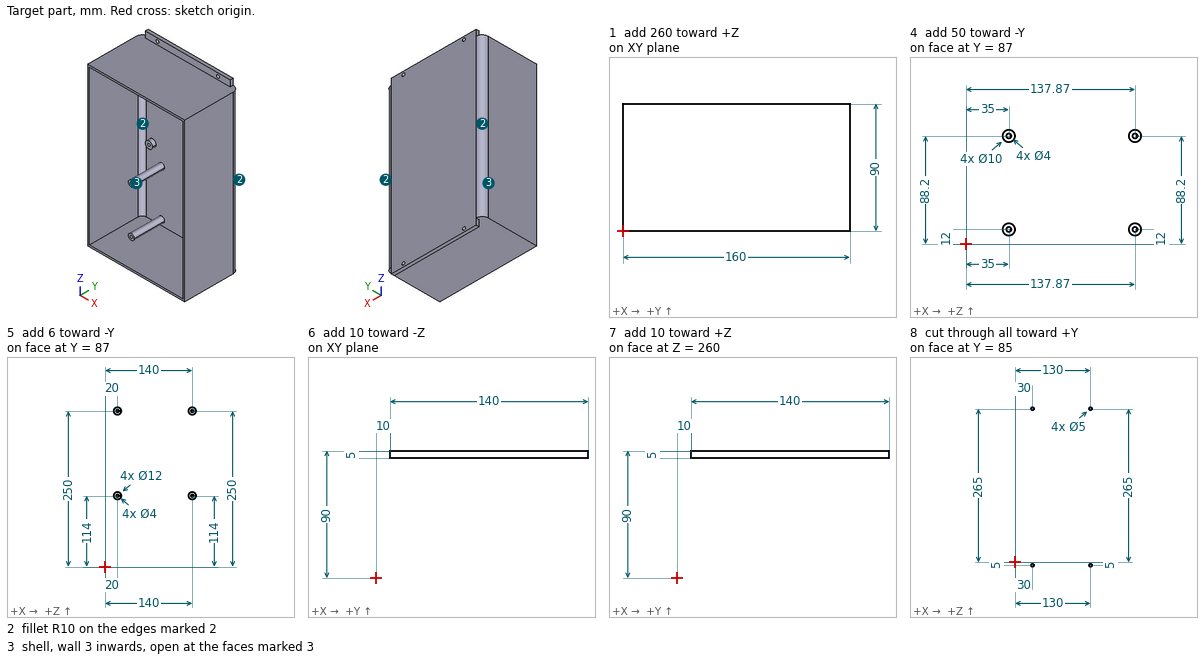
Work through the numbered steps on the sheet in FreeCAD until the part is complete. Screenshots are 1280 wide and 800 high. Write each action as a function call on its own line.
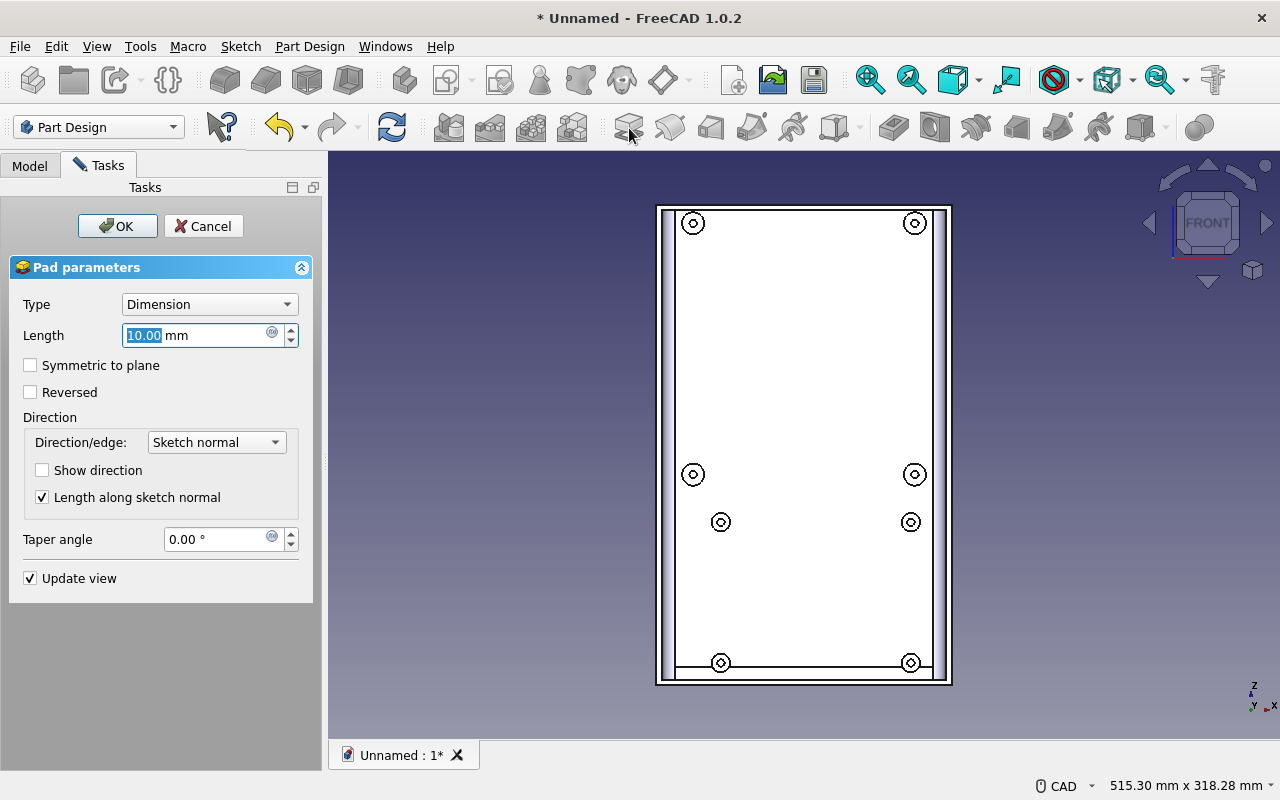
text(10)
key(Tab)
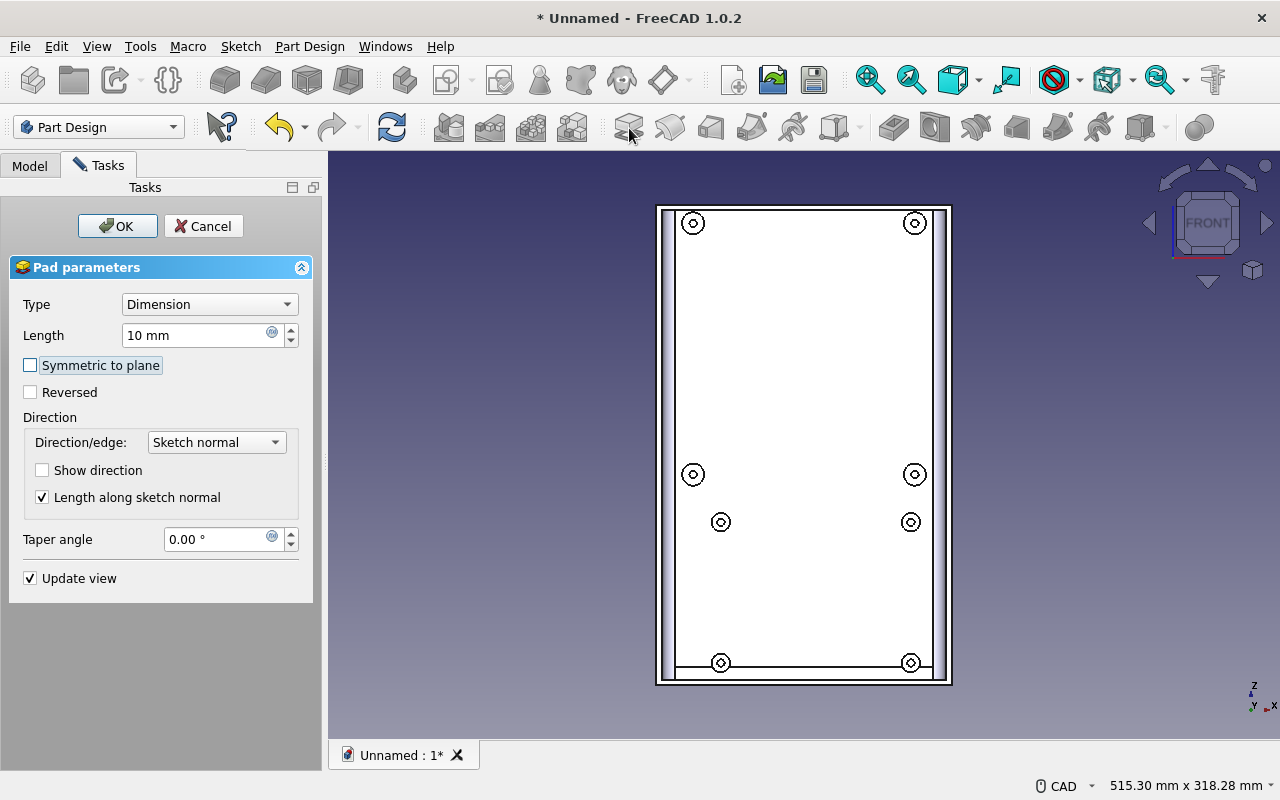
click(31, 392)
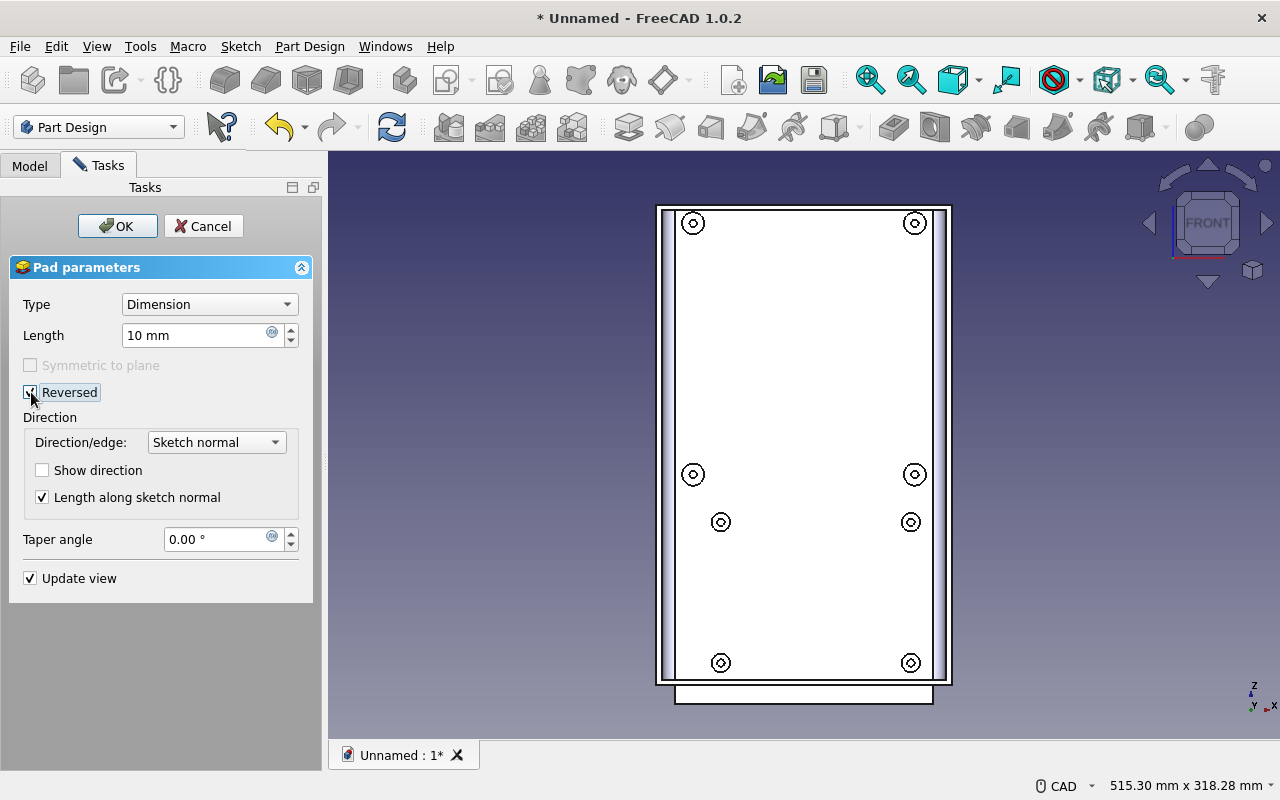
click(118, 226)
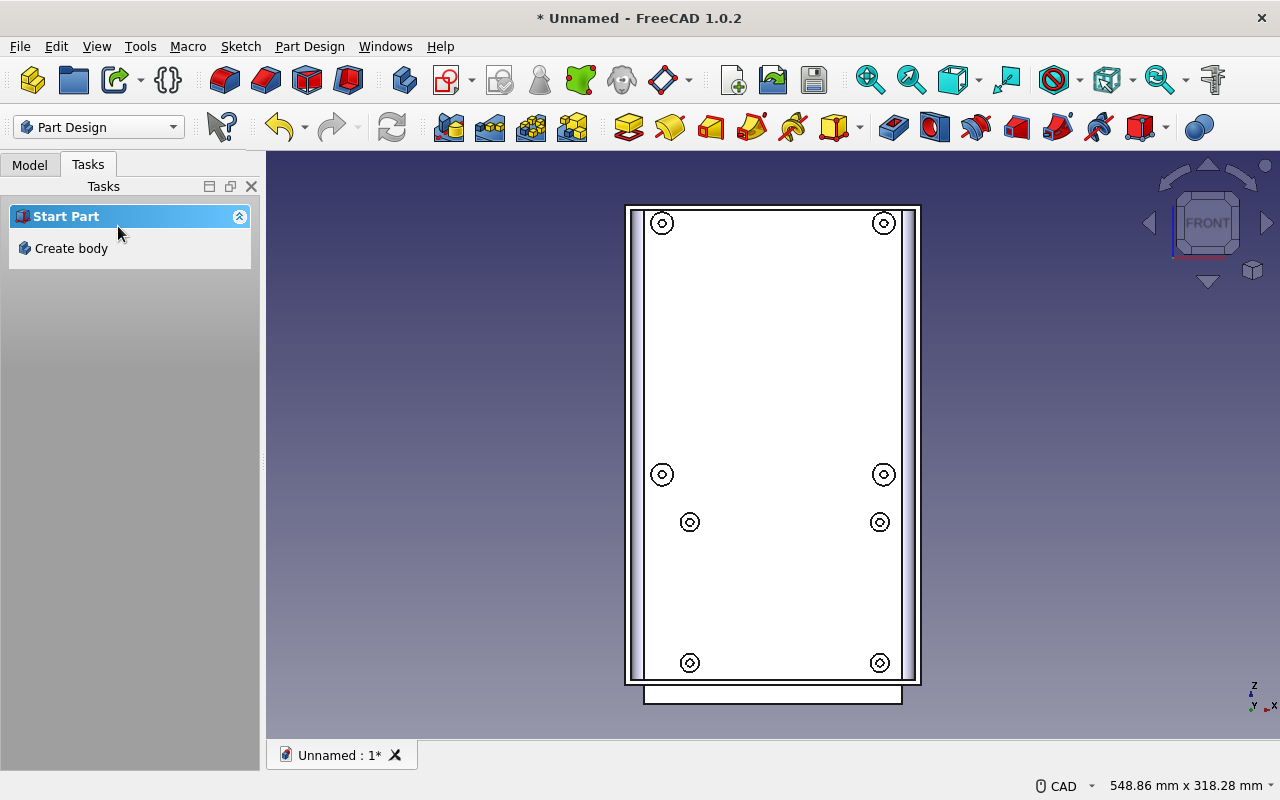
key(0)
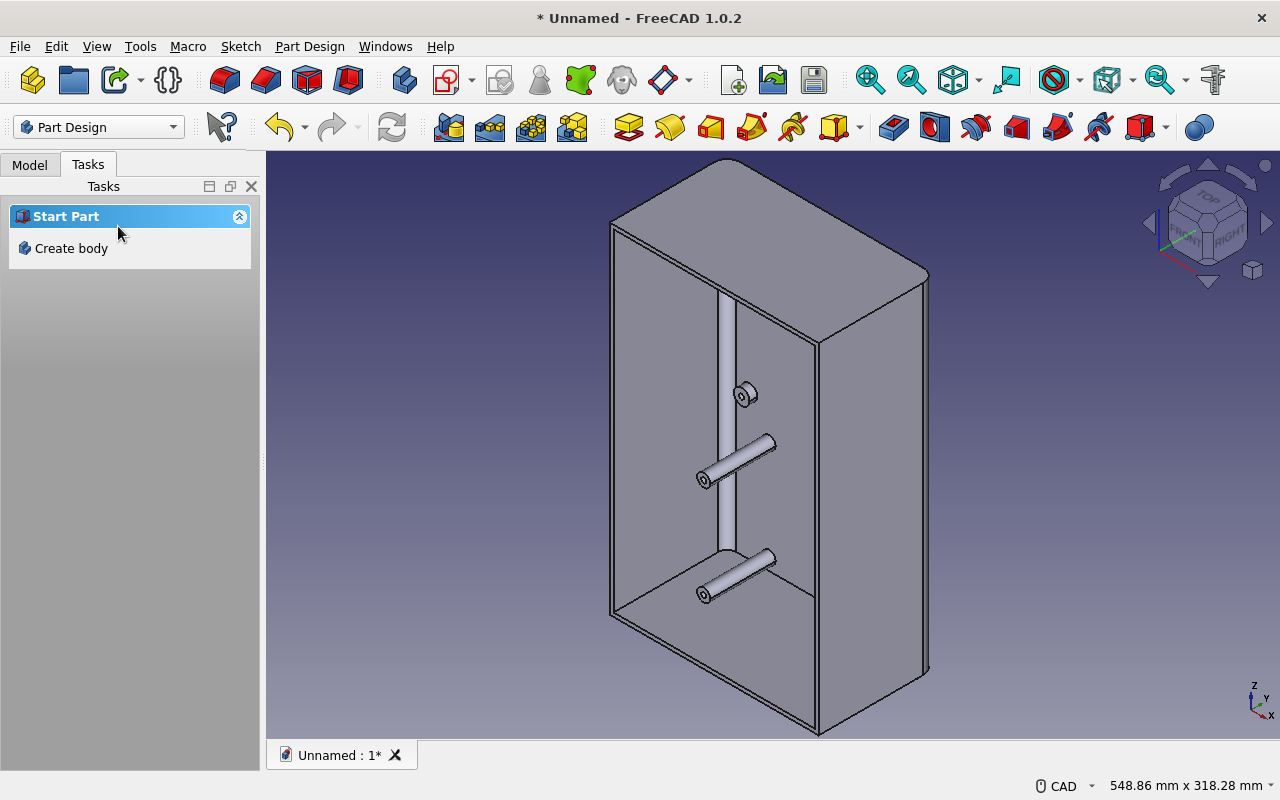
click(871, 80)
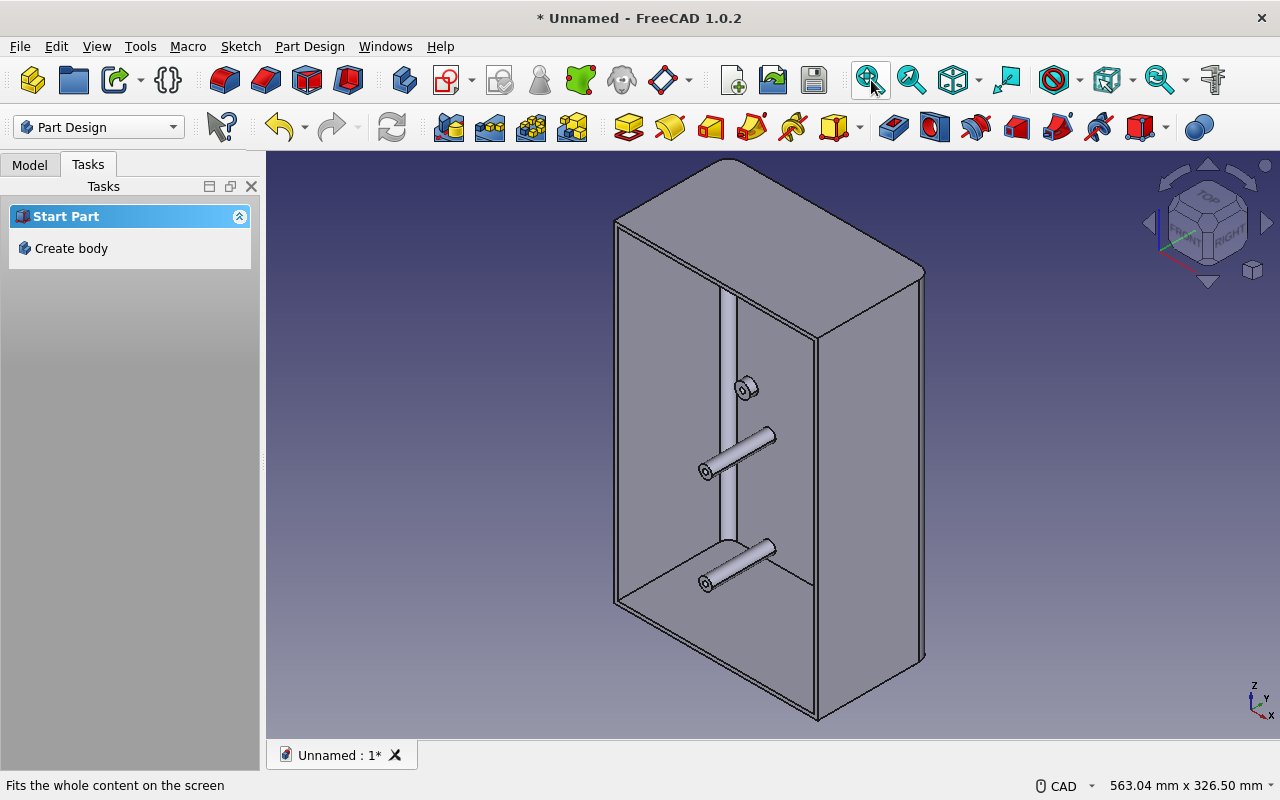
click(802, 262)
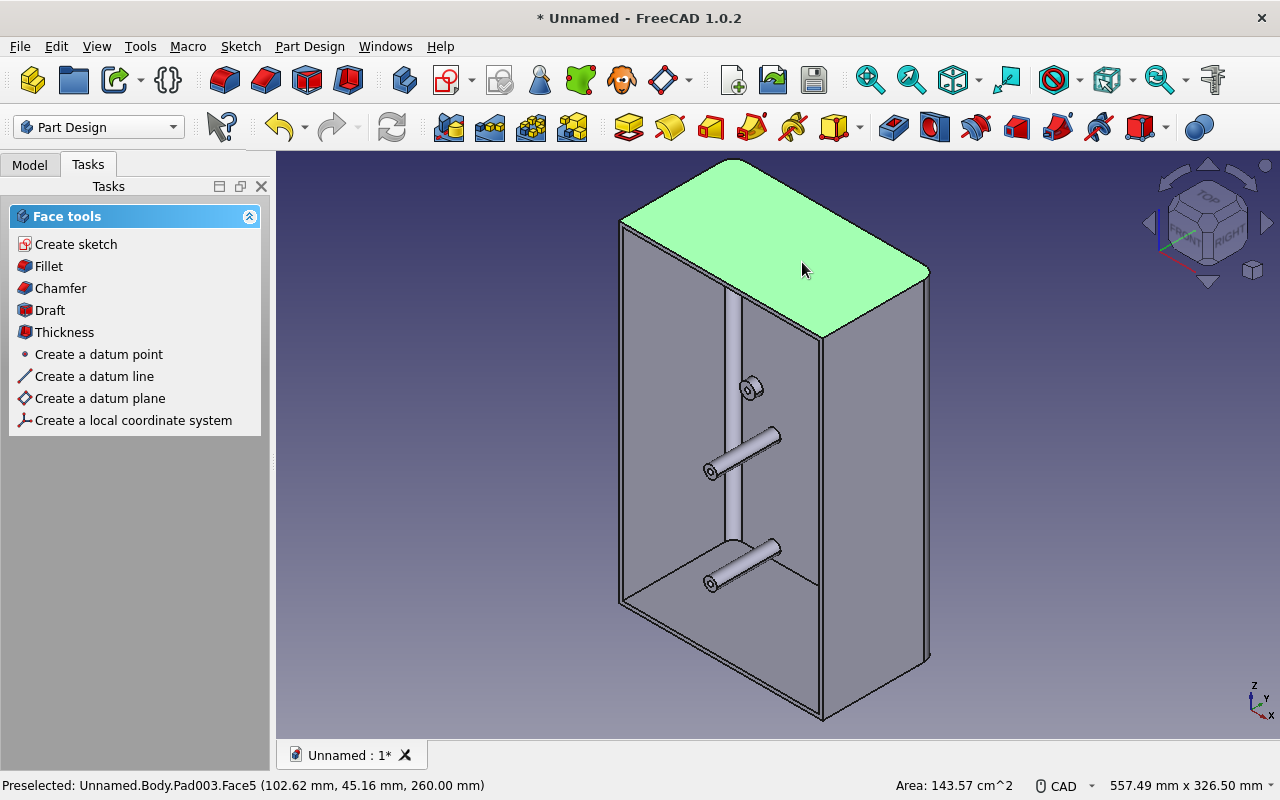
click(446, 80)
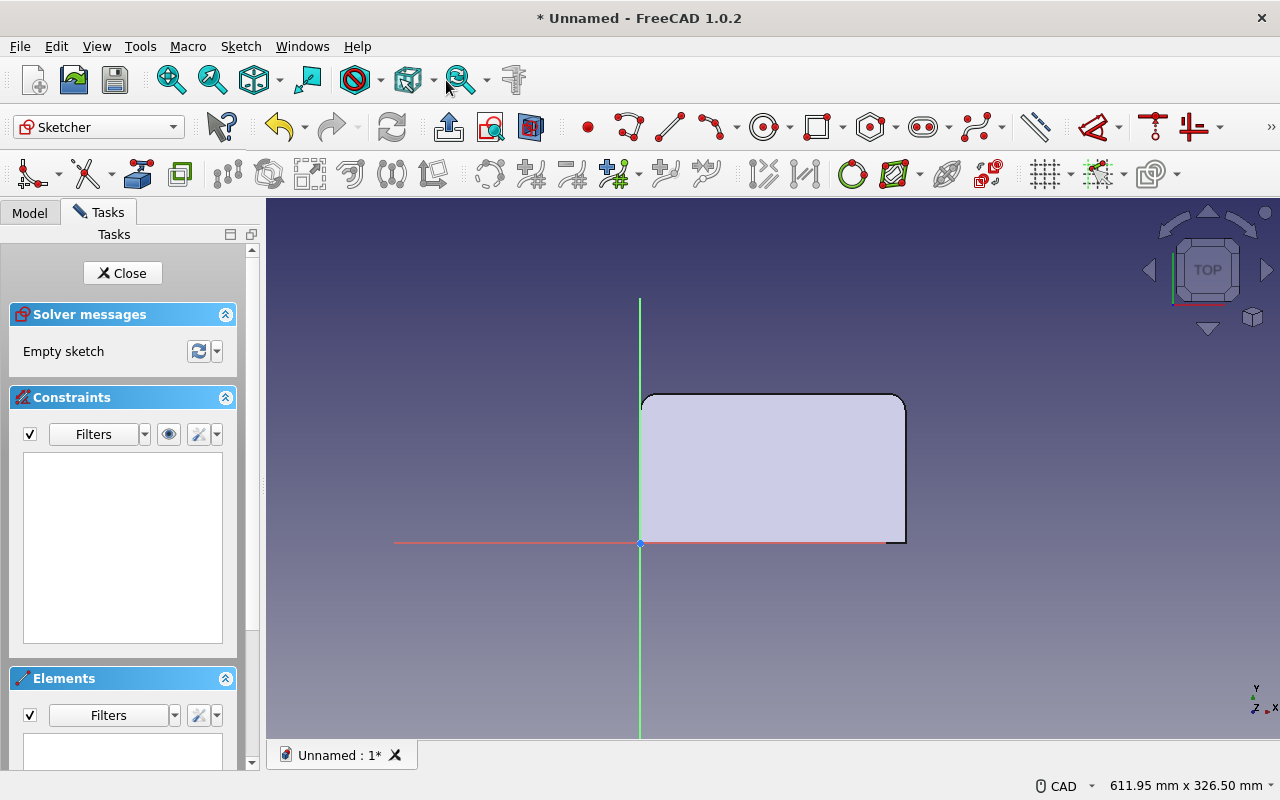
scroll(814, 469, up, 4)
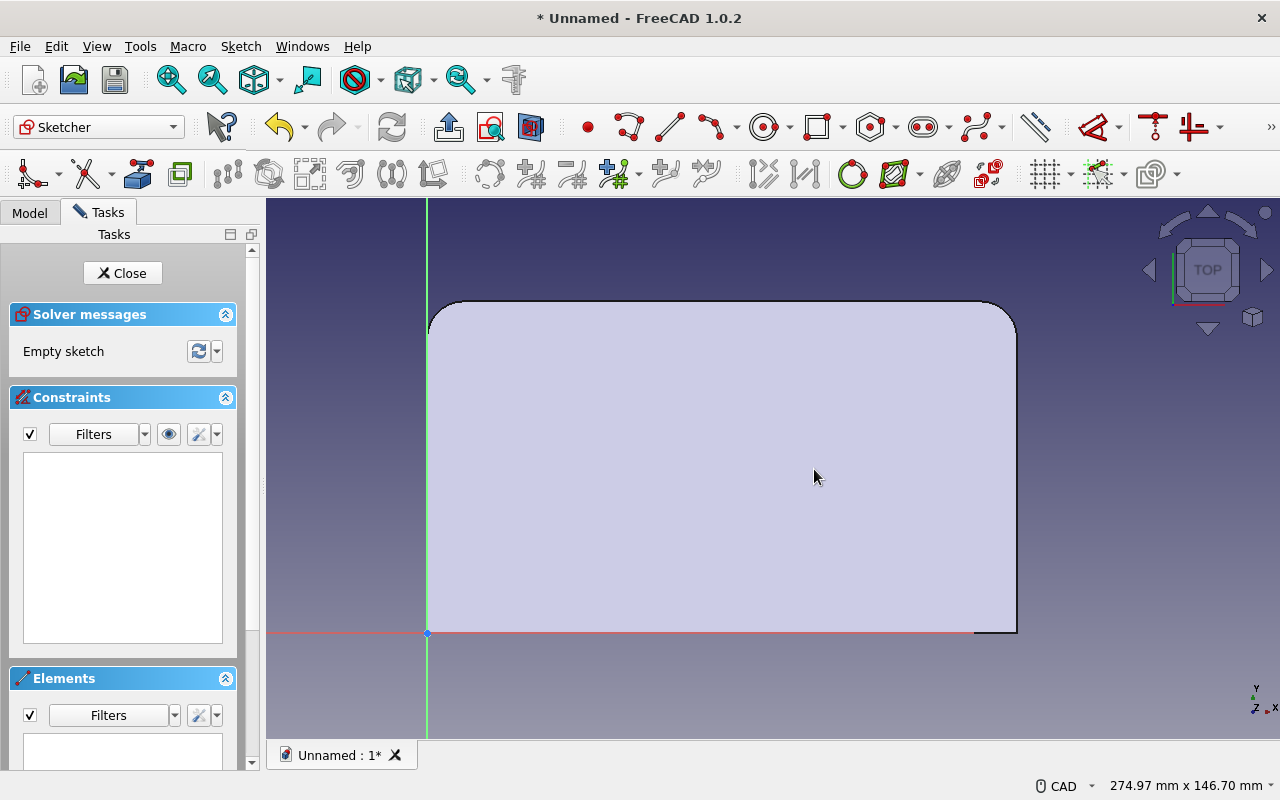
click(816, 128)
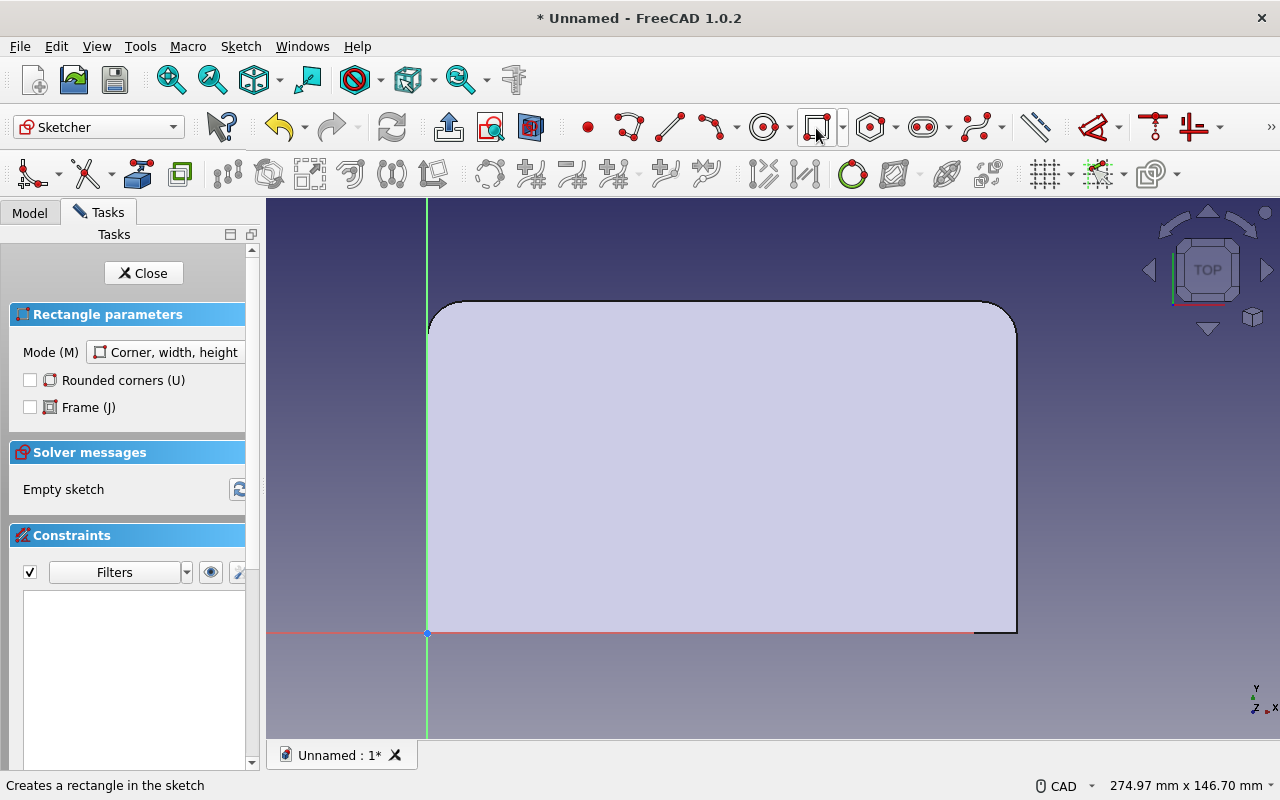
click(464, 301)
click(980, 320)
key(Escape)